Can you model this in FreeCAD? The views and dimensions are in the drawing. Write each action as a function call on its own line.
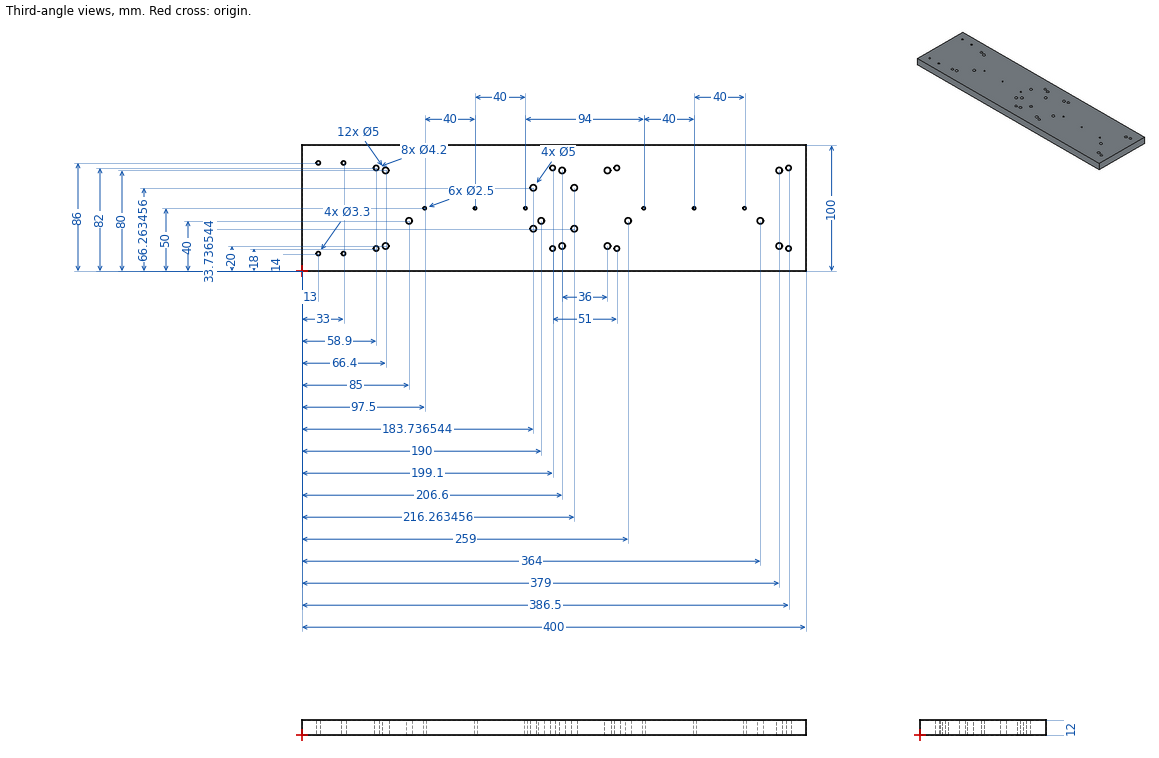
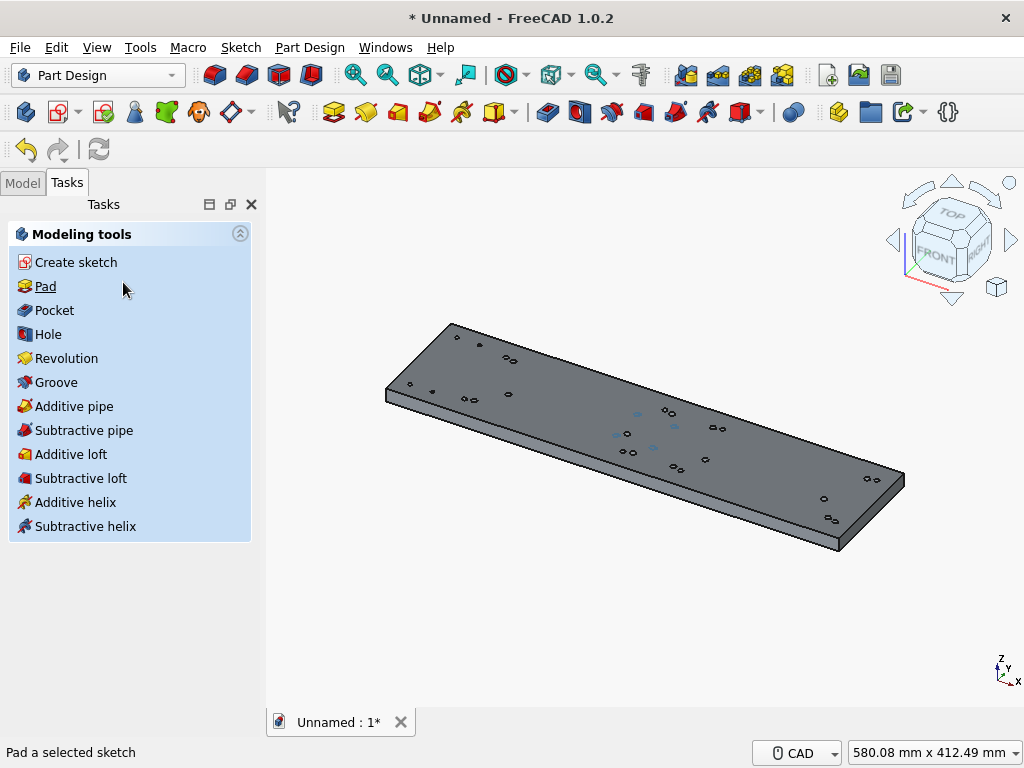
click(548, 112)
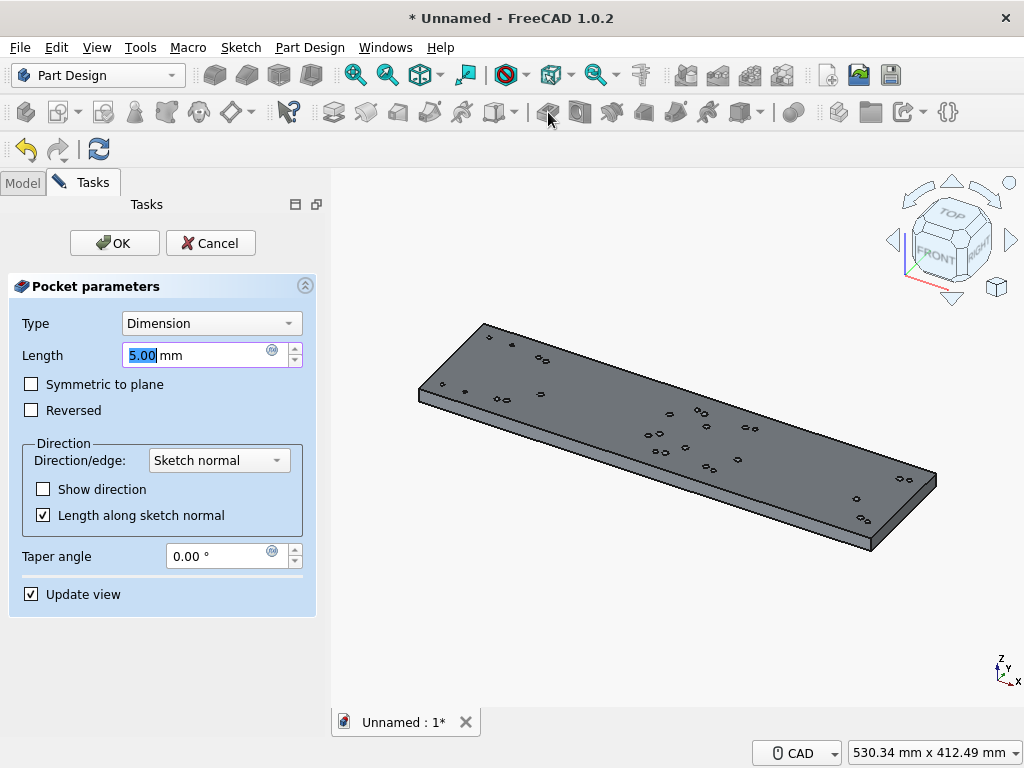
click(212, 324)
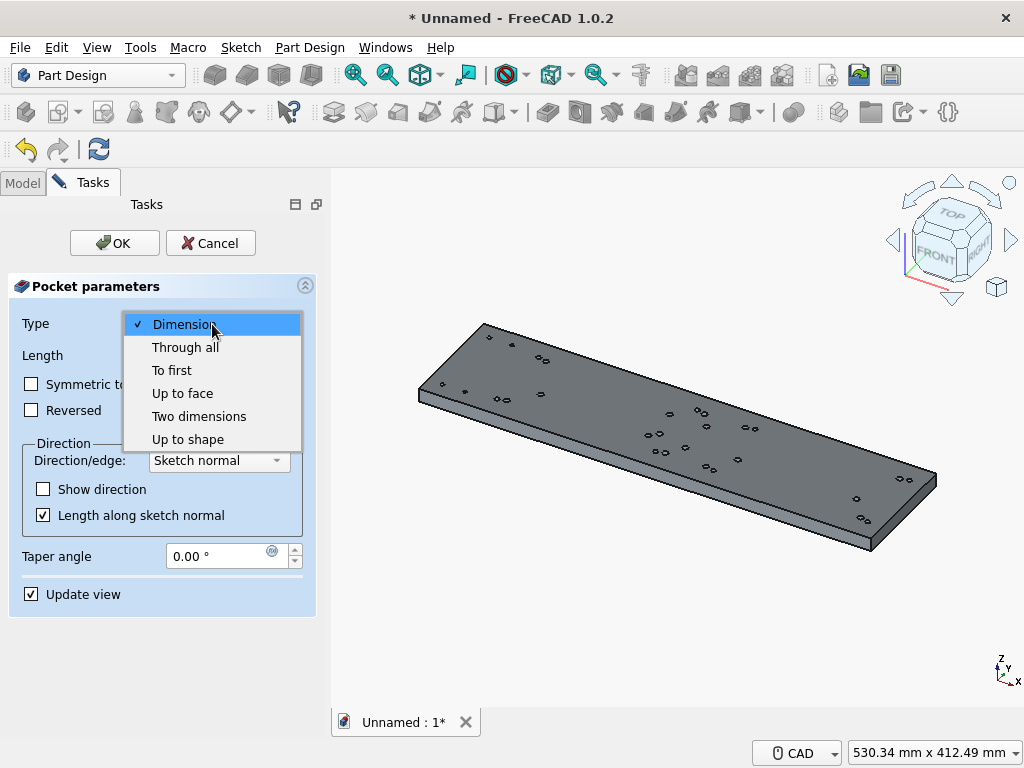
click(212, 348)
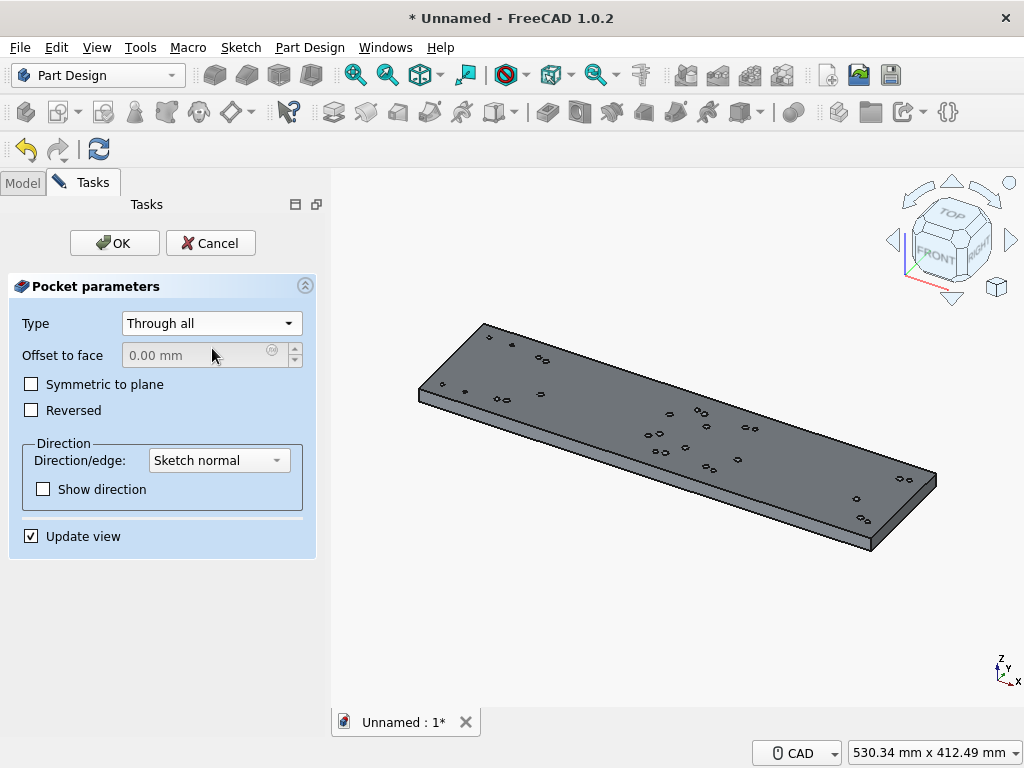
click(115, 243)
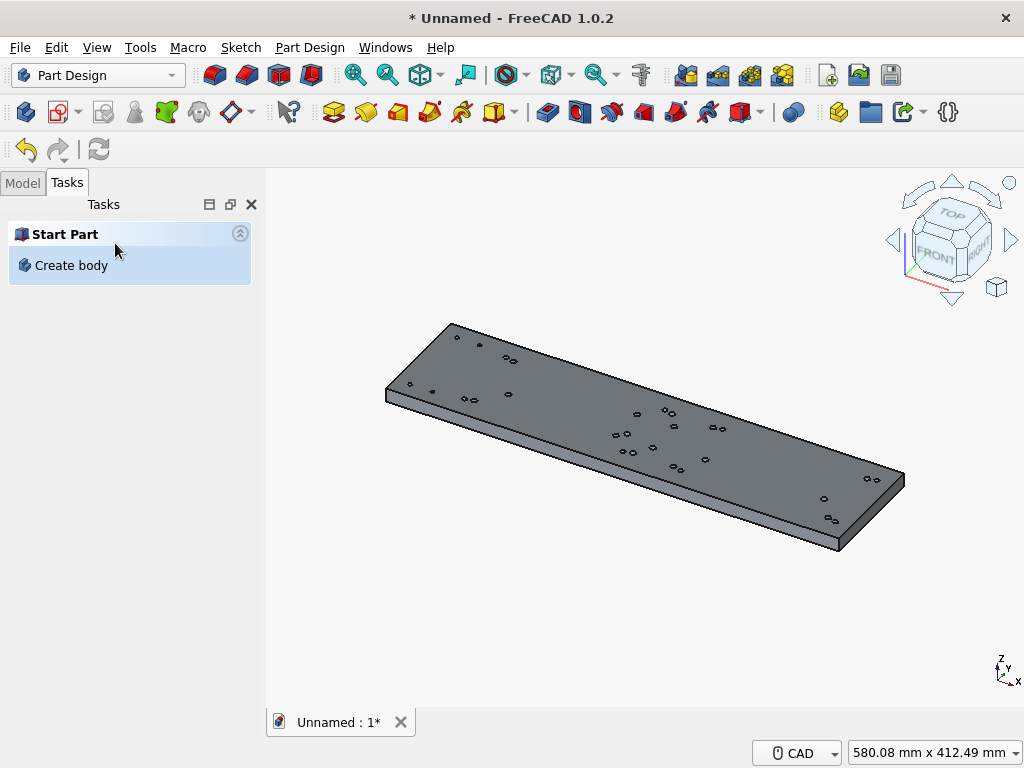
click(774, 473)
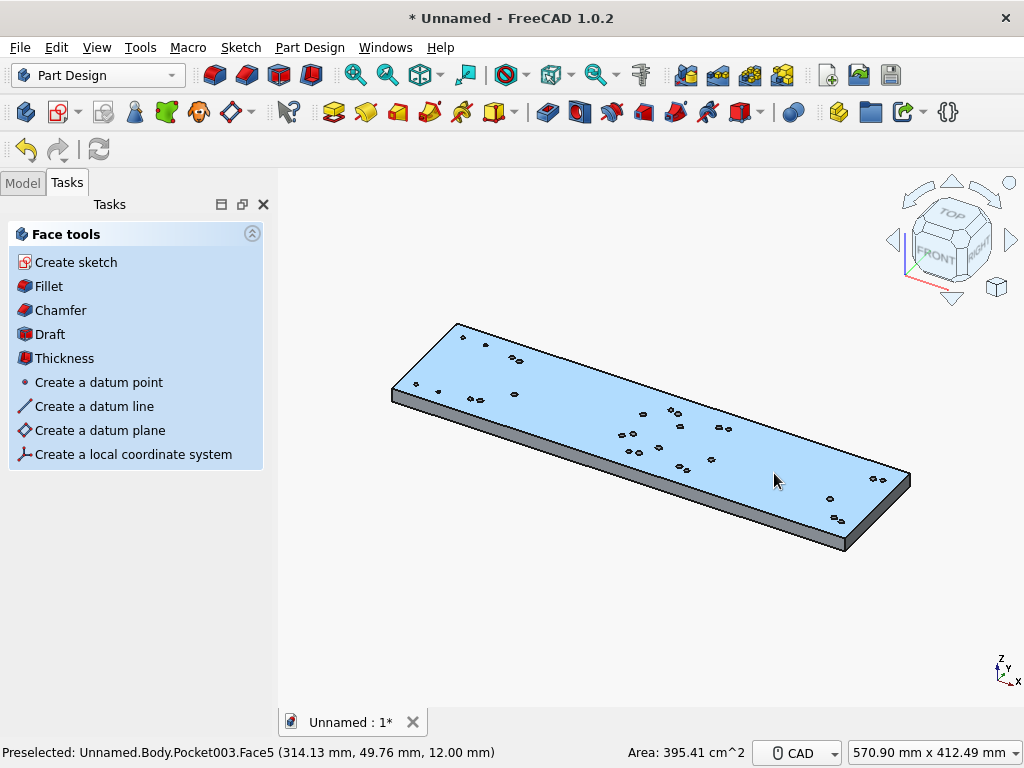
click(58, 112)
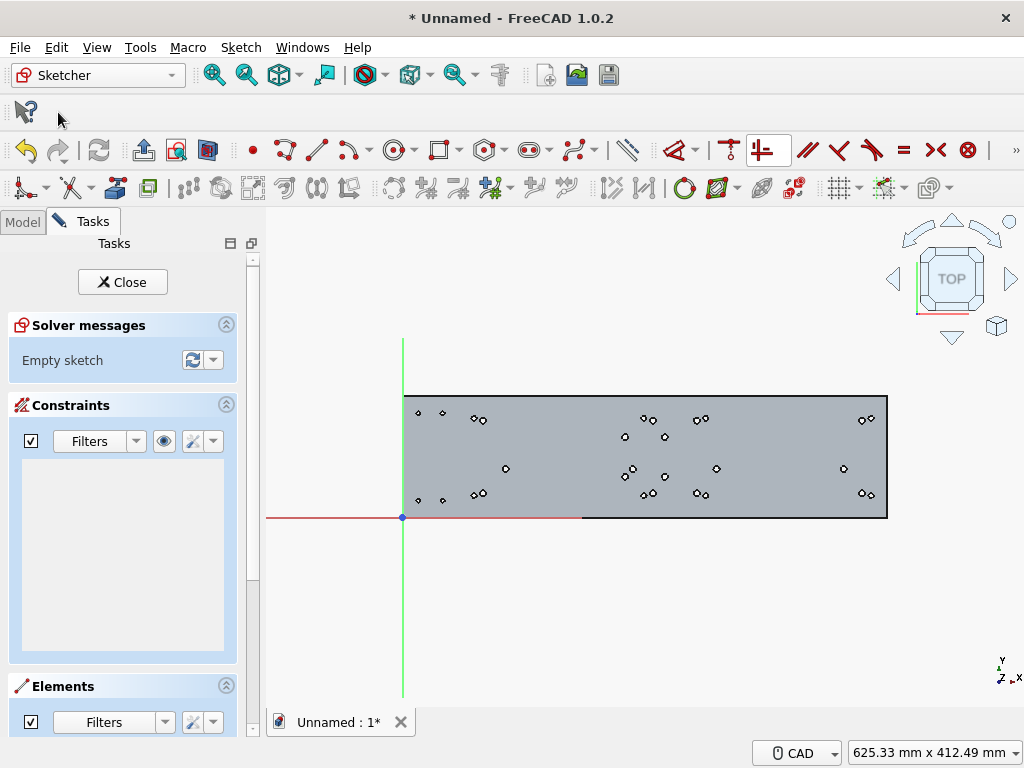
click(394, 150)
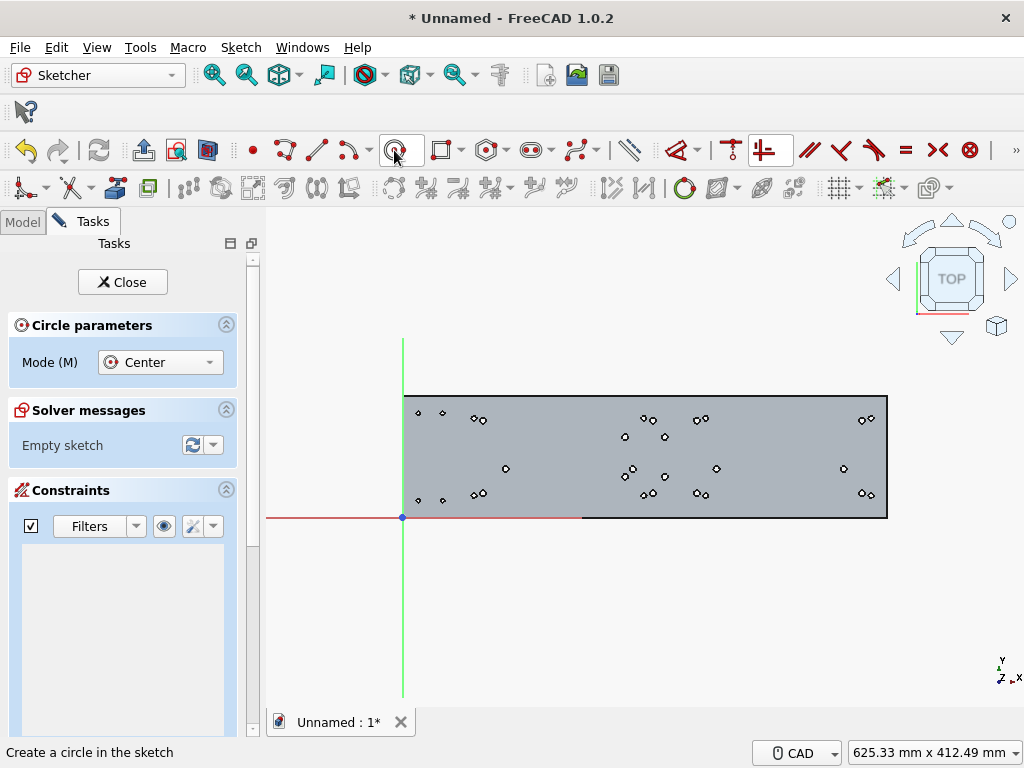
scroll(521, 457, up, 14)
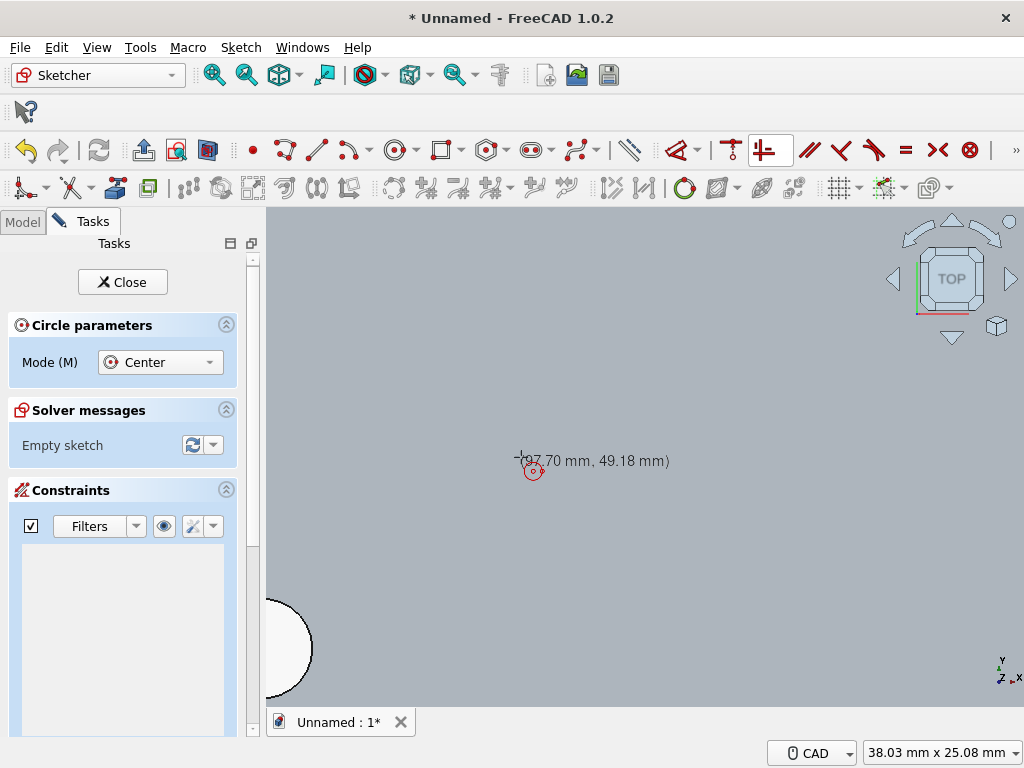
scroll(479, 426, down, 14)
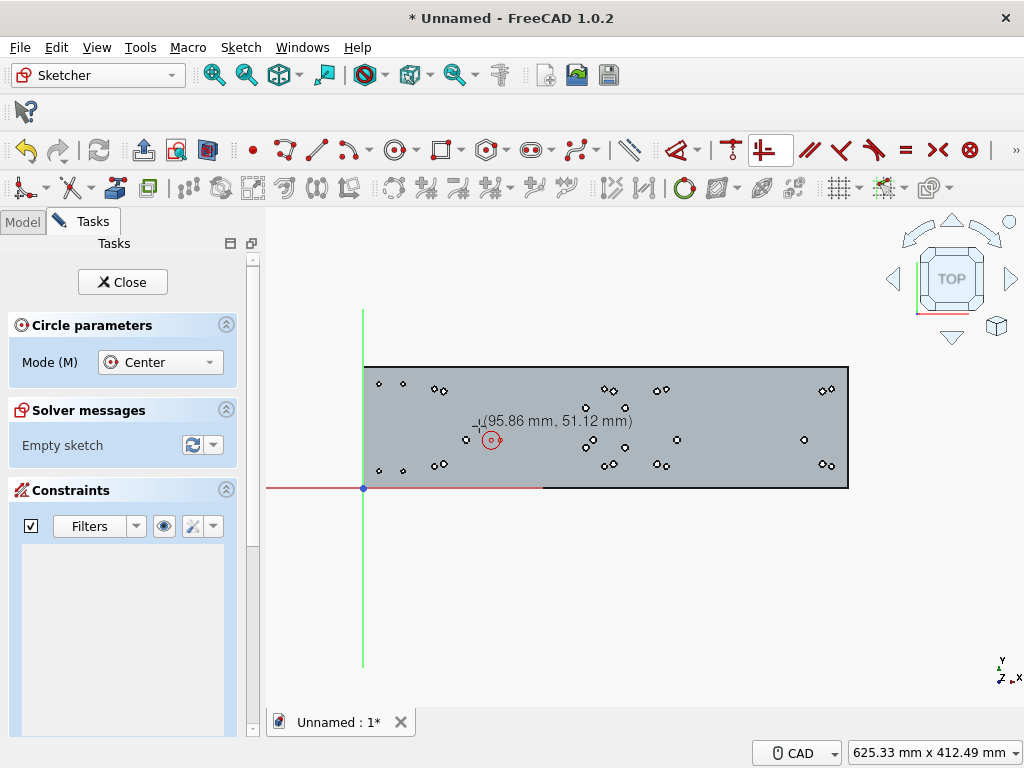
click(481, 428)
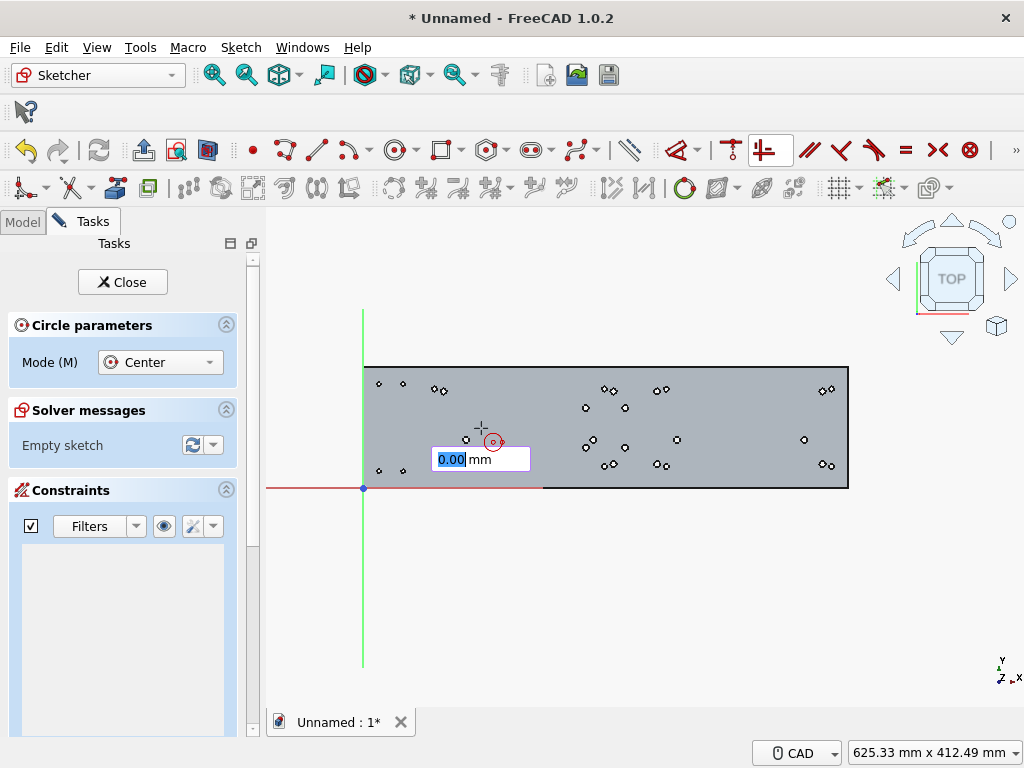
scroll(482, 427, up, 12)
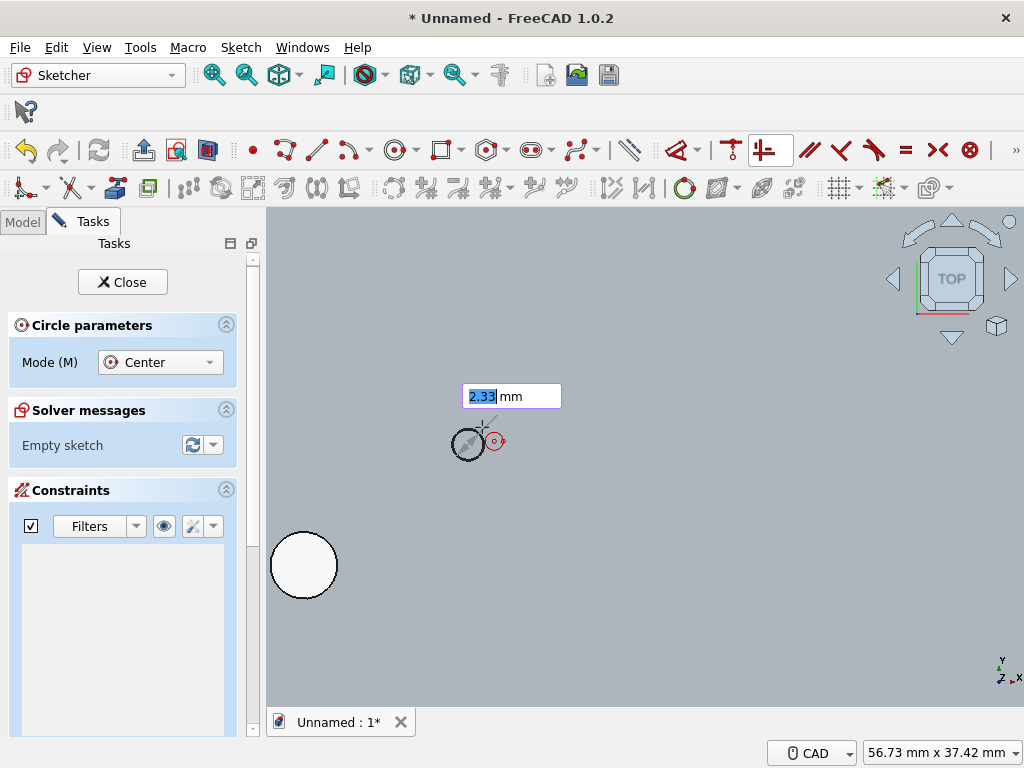
click(483, 420)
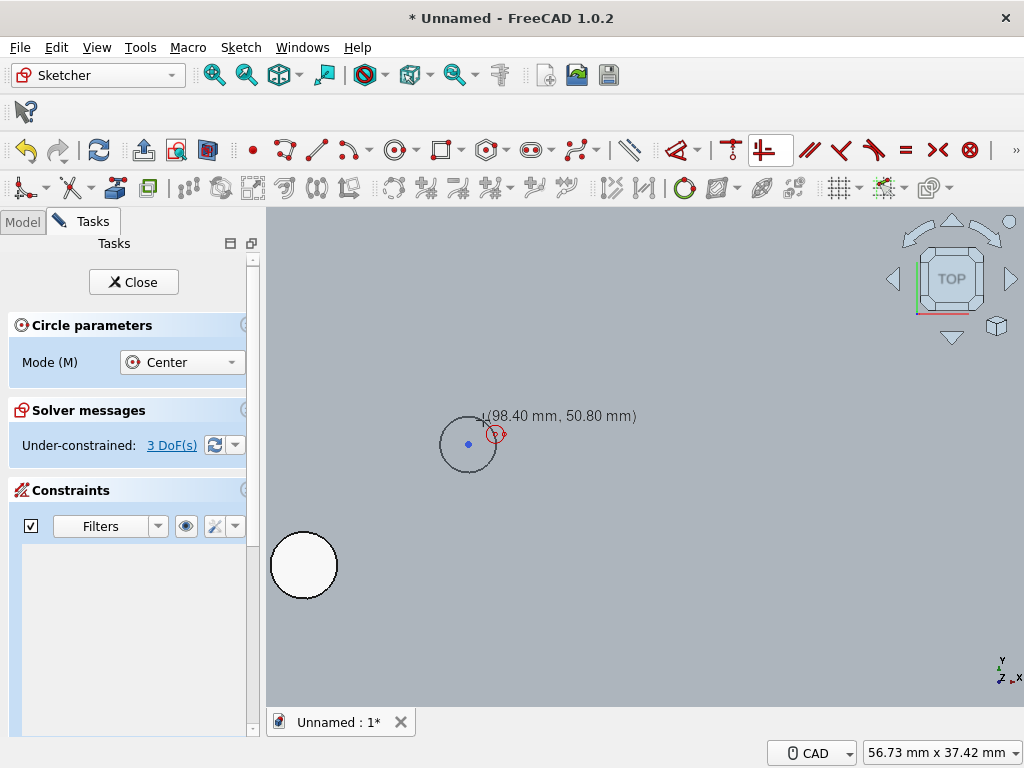
scroll(482, 427, down, 12)